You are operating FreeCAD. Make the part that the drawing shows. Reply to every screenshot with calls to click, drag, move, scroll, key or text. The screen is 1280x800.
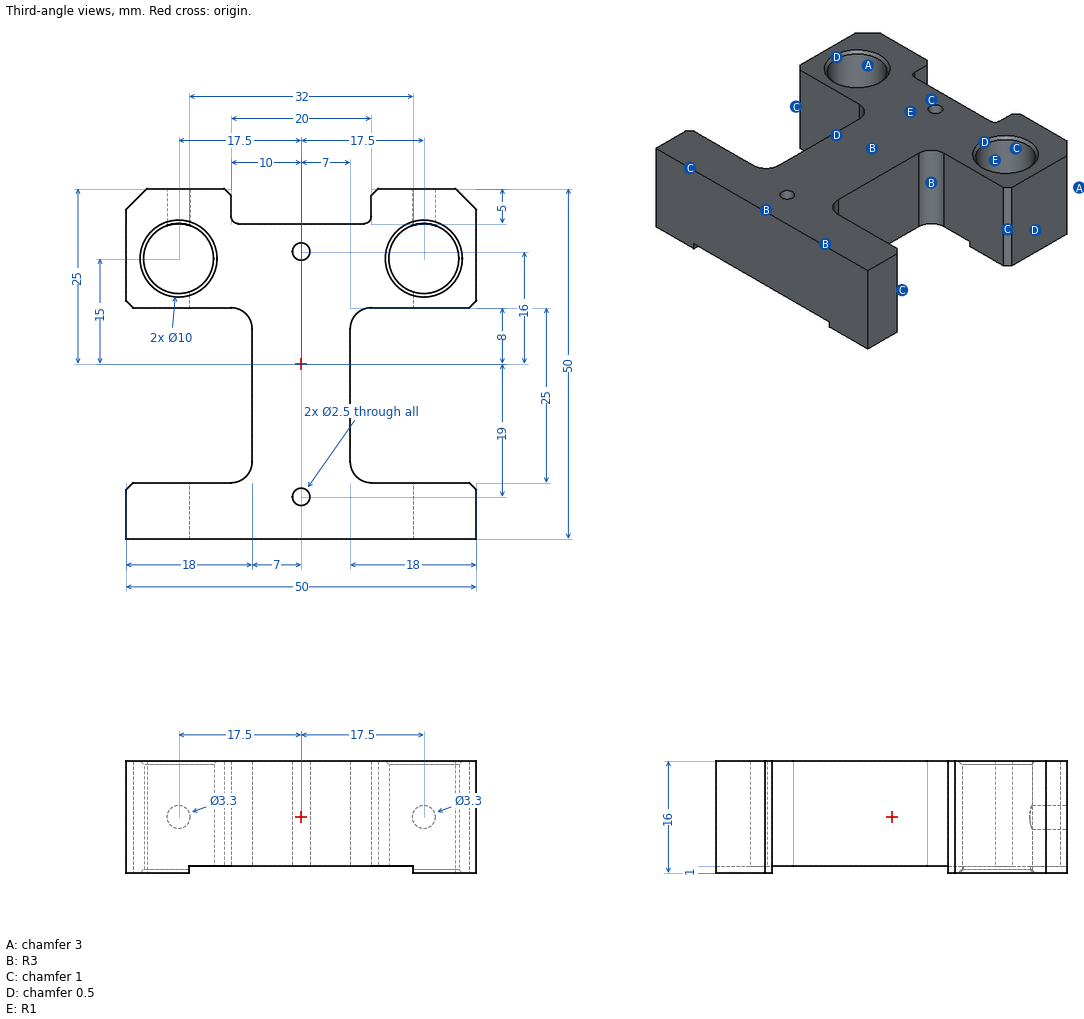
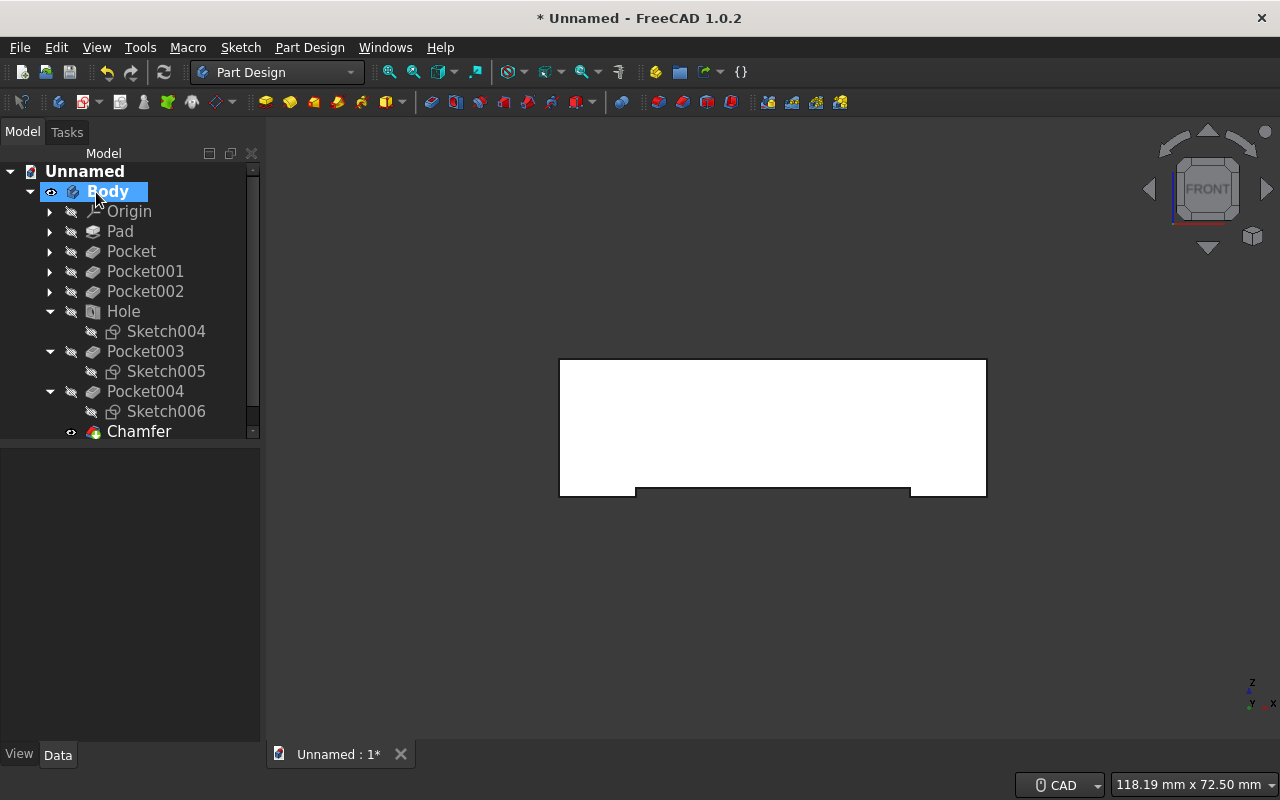
click(390, 72)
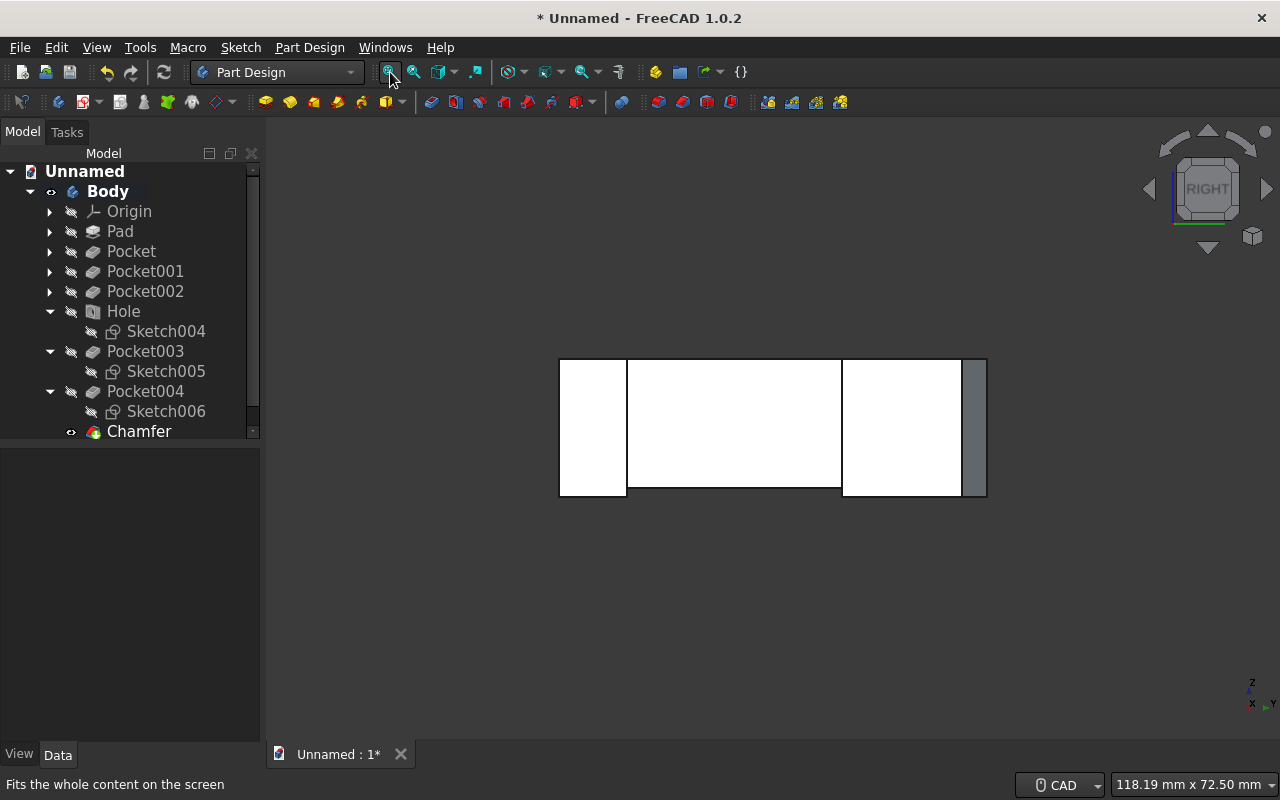
key(5)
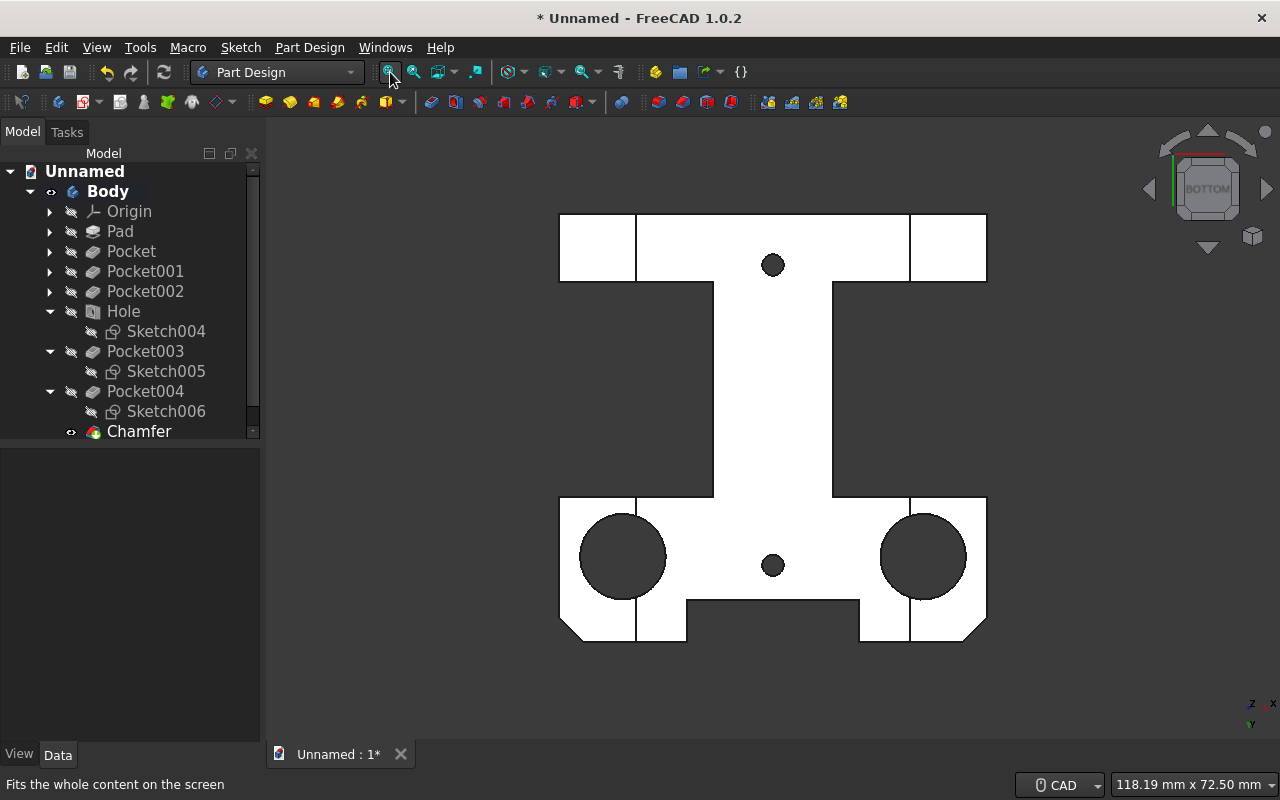
key(4)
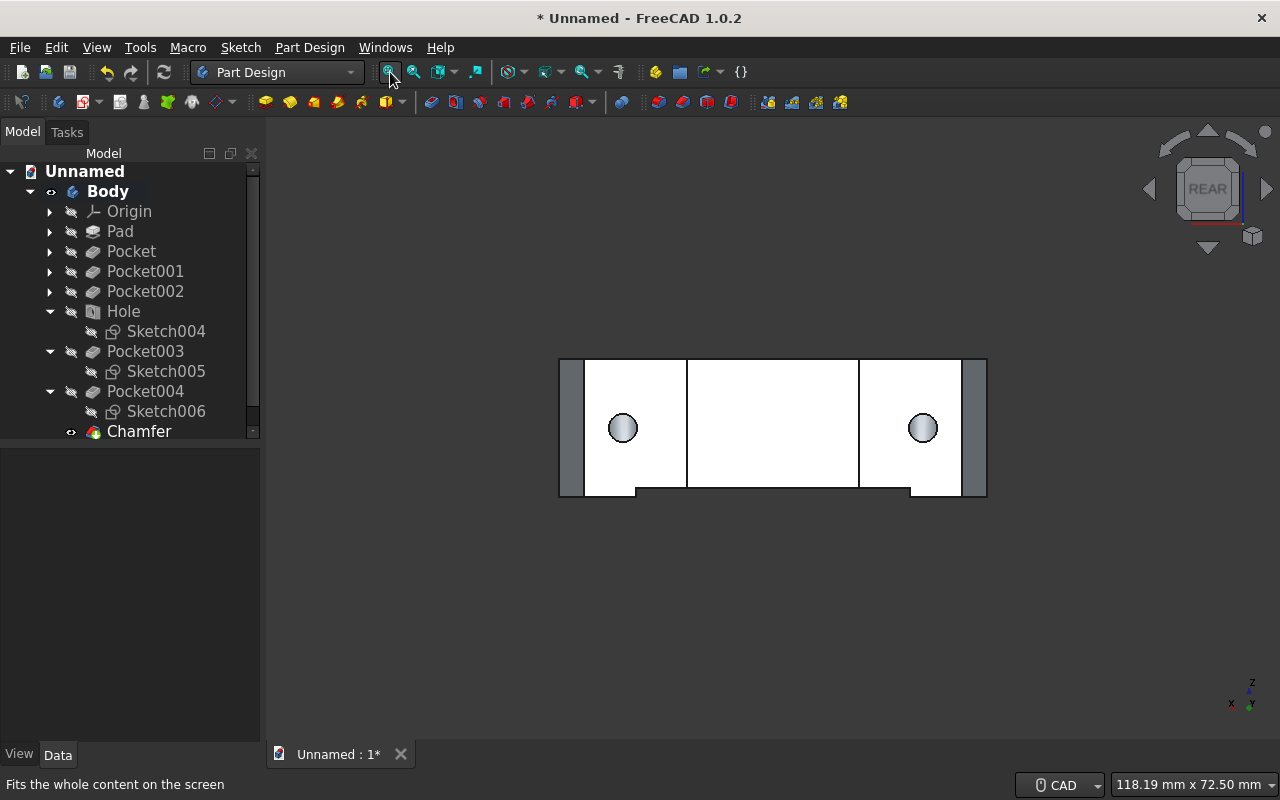
click(390, 72)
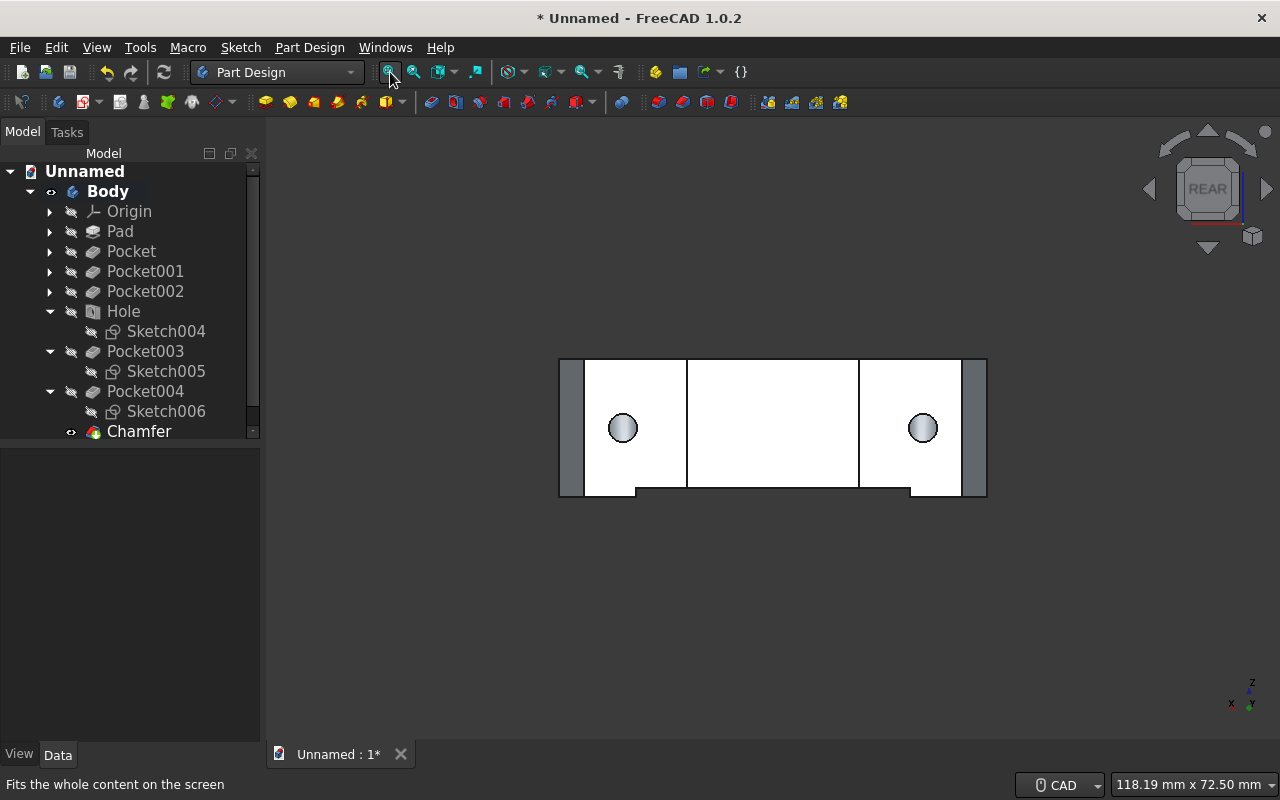
key(6)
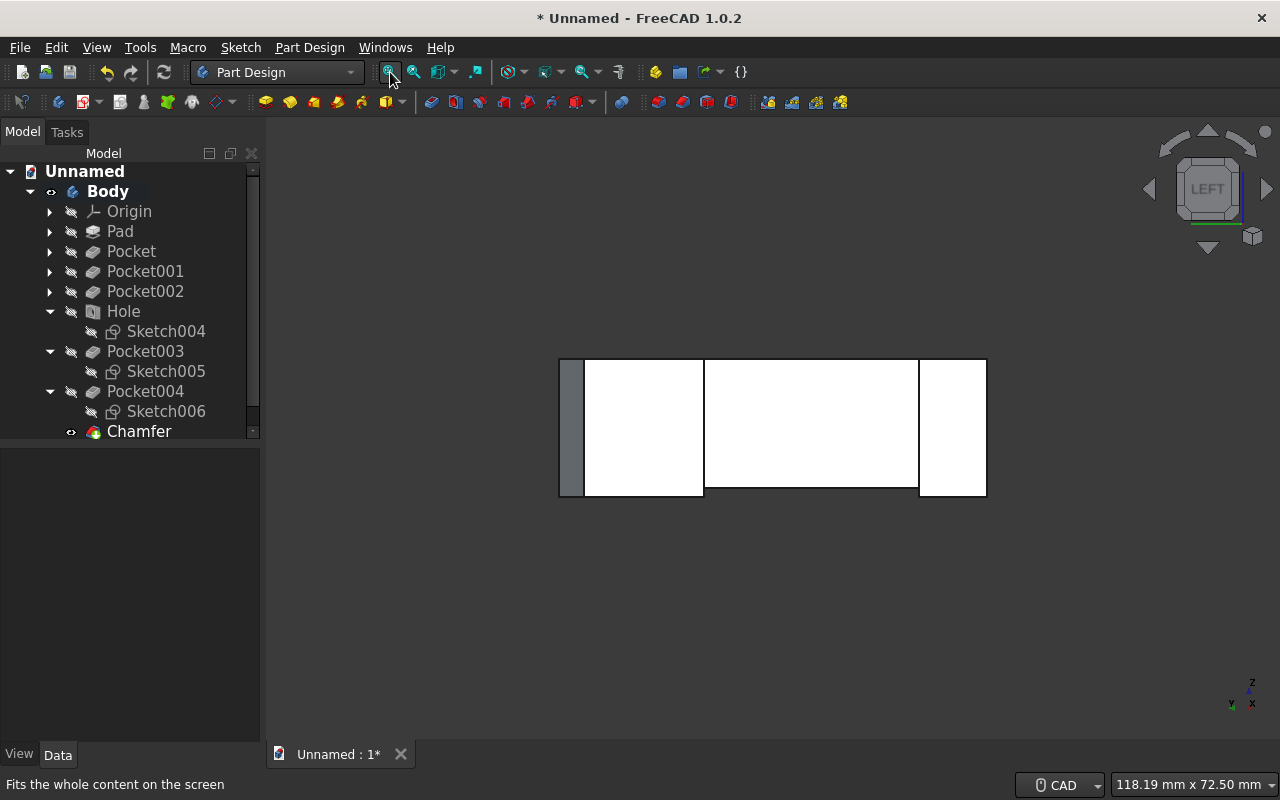
key(v)
key(f)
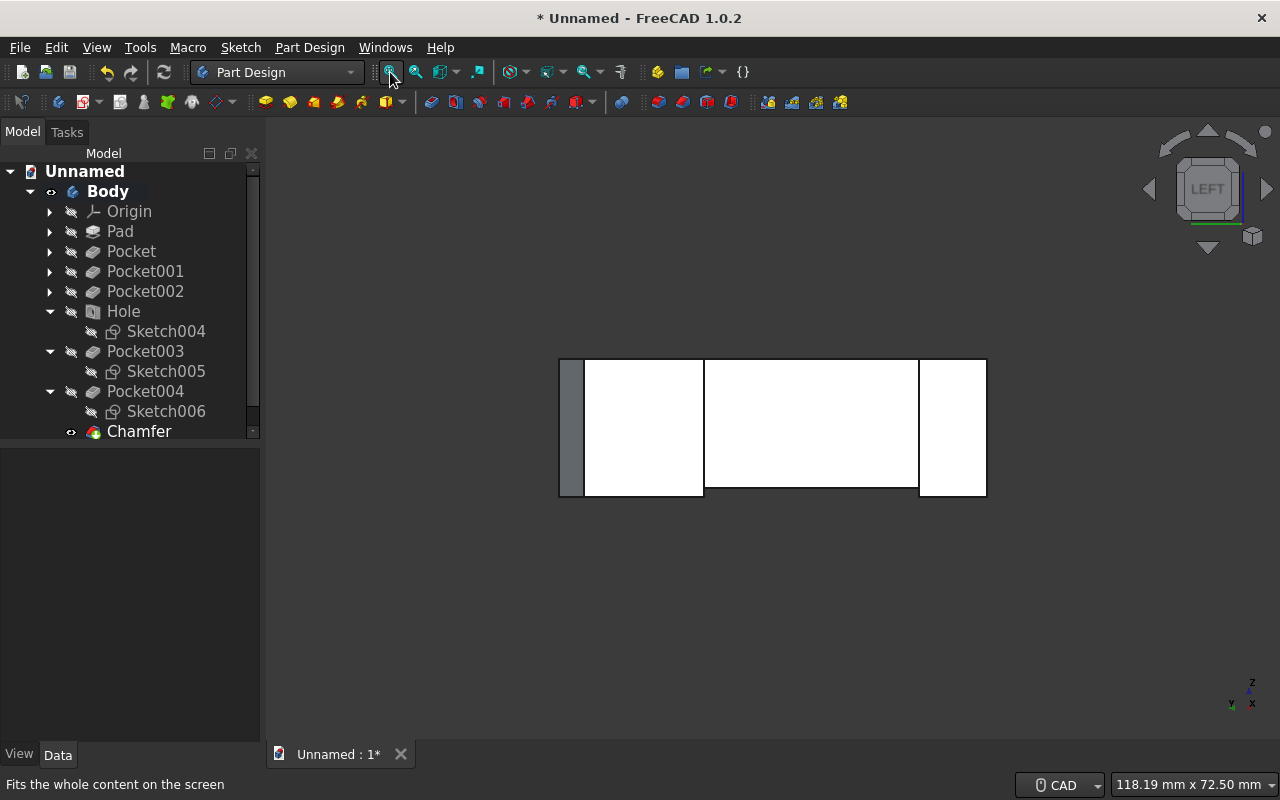
key(v)
key(3)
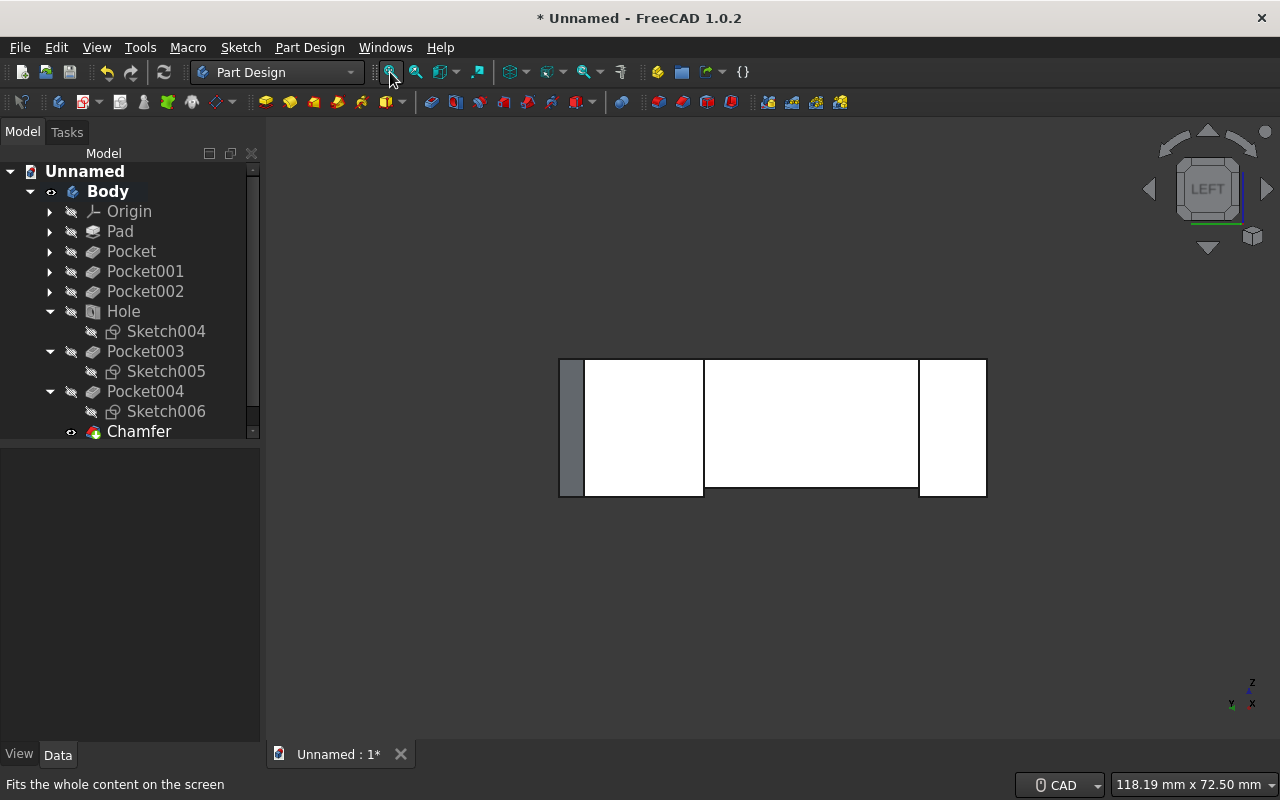
key(0)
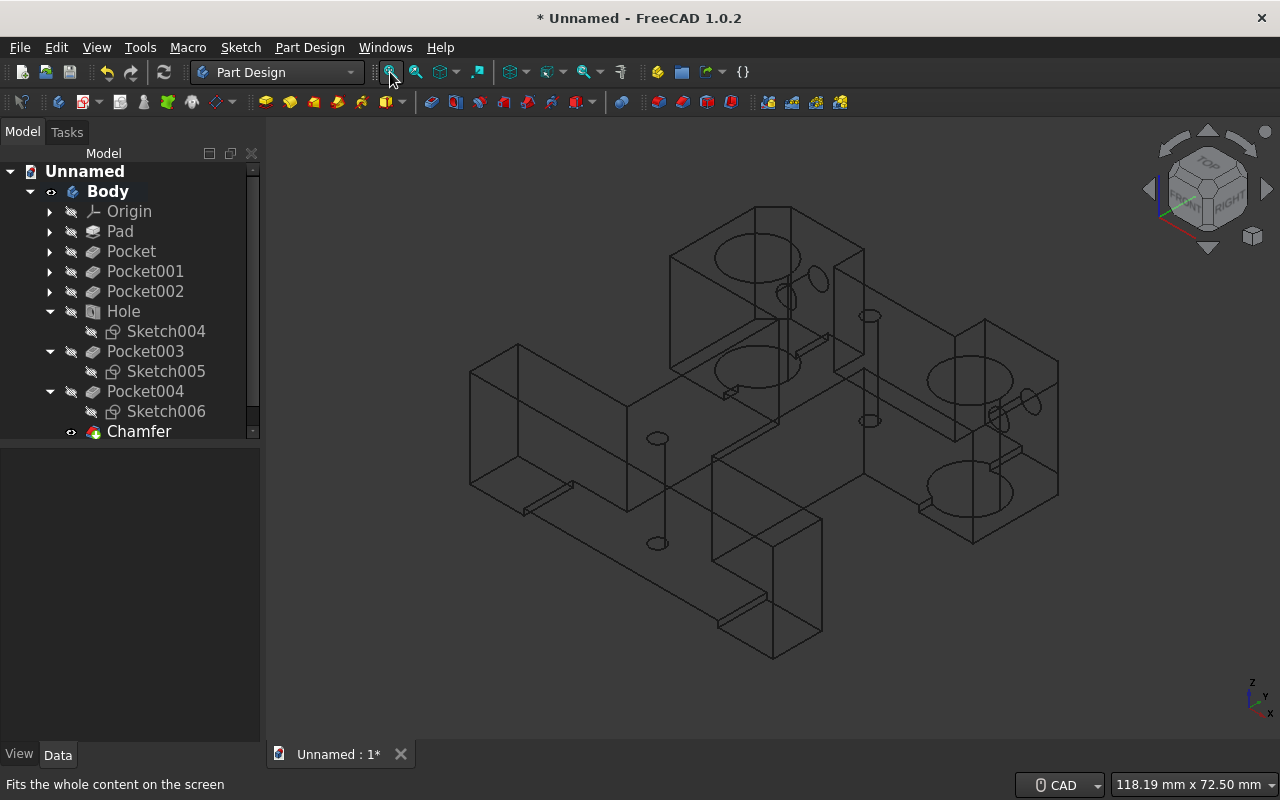
click(627, 448)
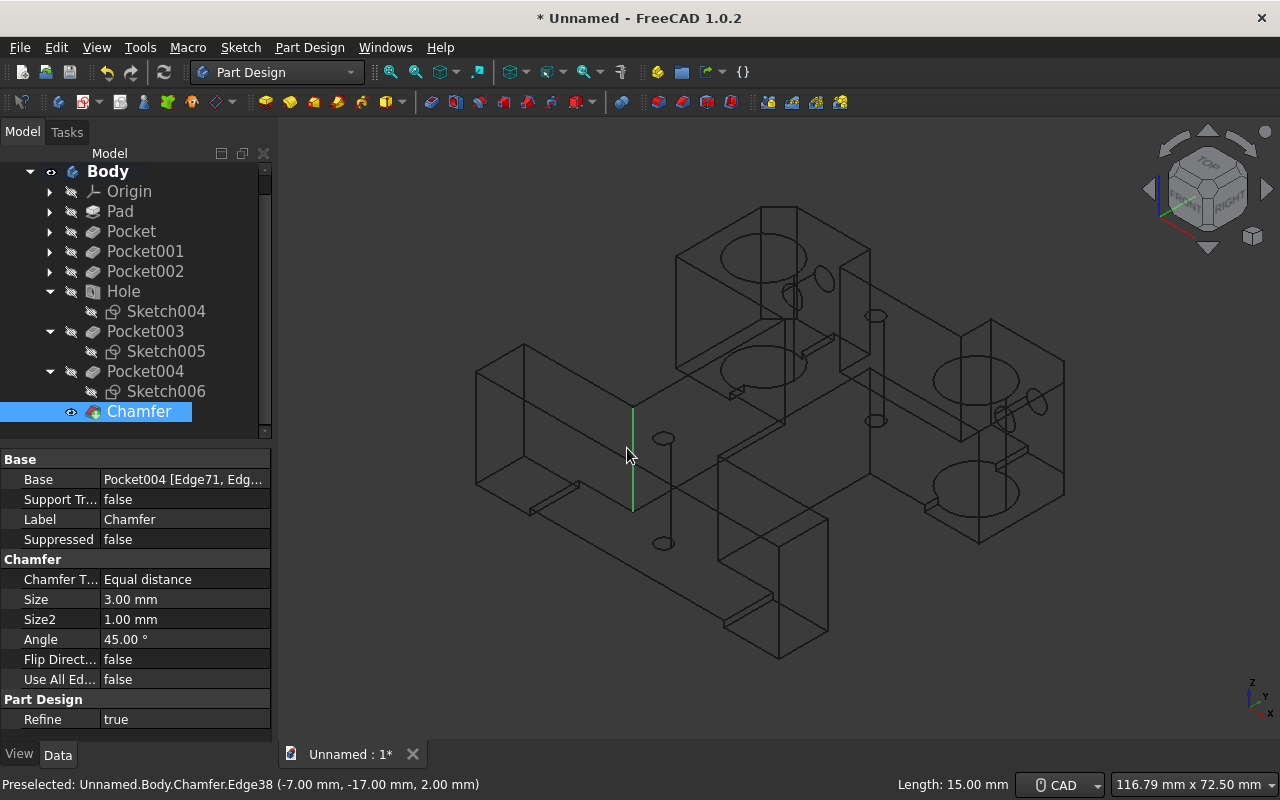
click(785, 371, ctrl)